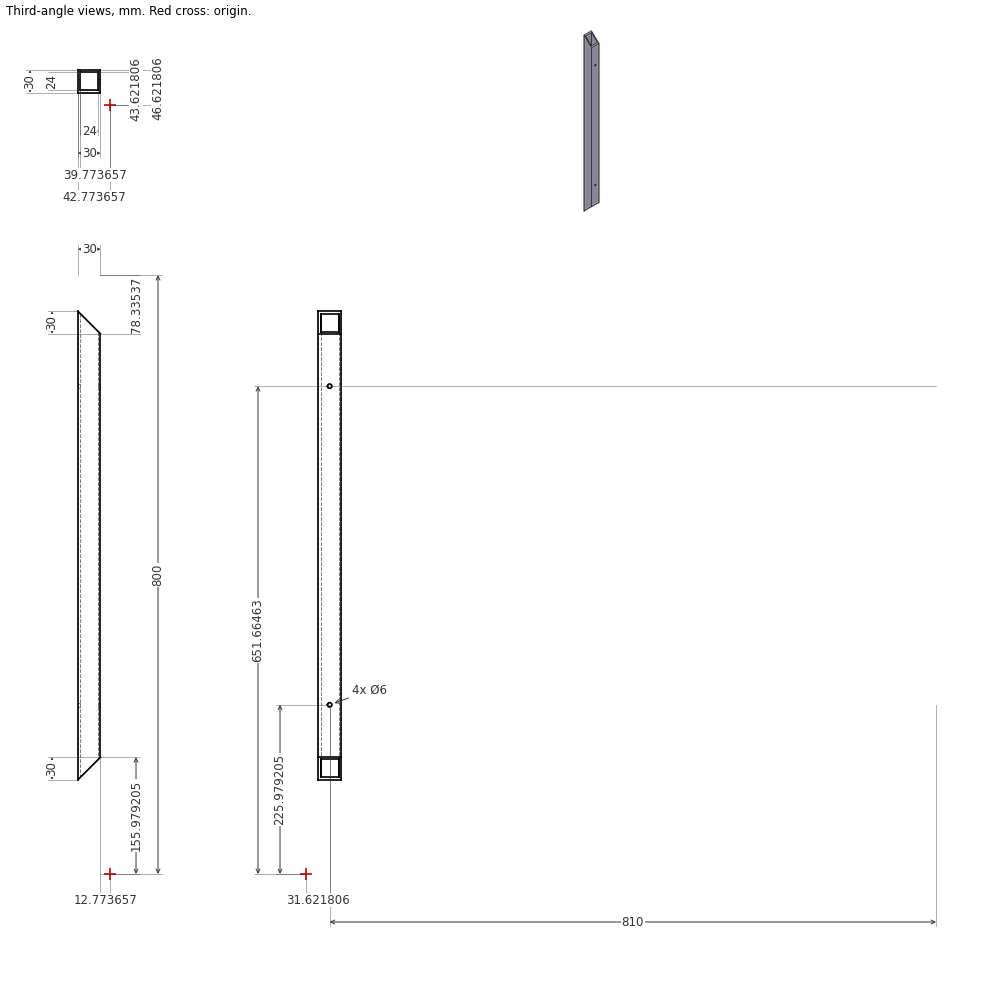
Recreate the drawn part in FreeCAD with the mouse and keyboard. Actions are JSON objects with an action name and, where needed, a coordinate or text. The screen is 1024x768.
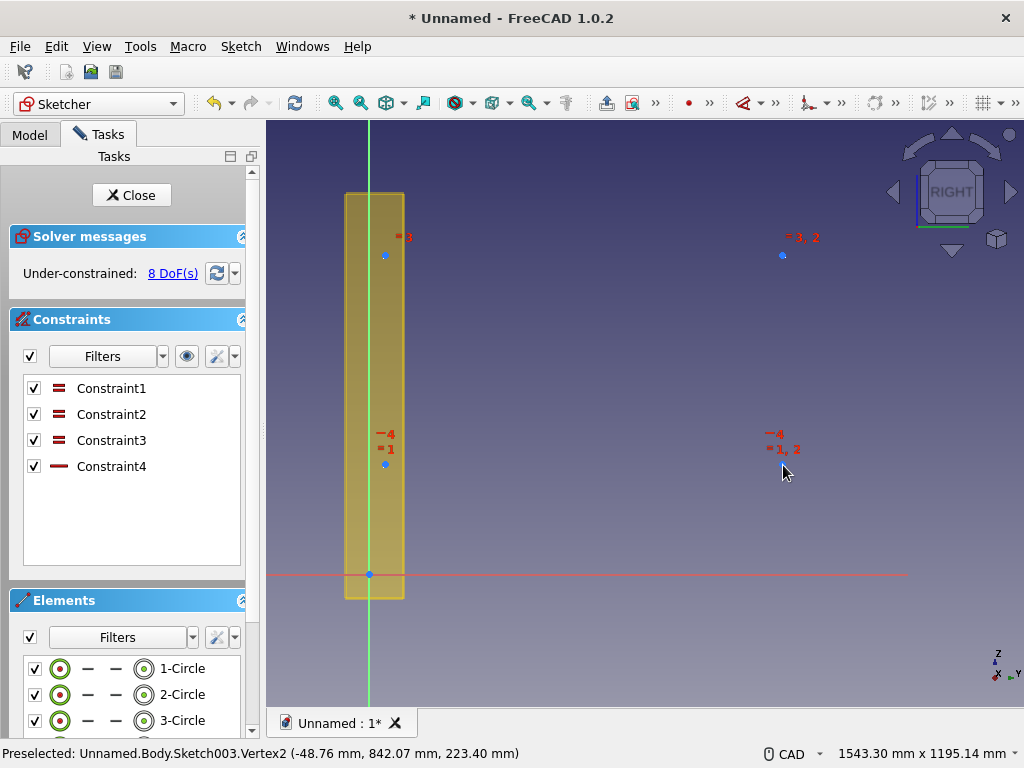
{"action": "left_click", "coordinate": [783, 465]}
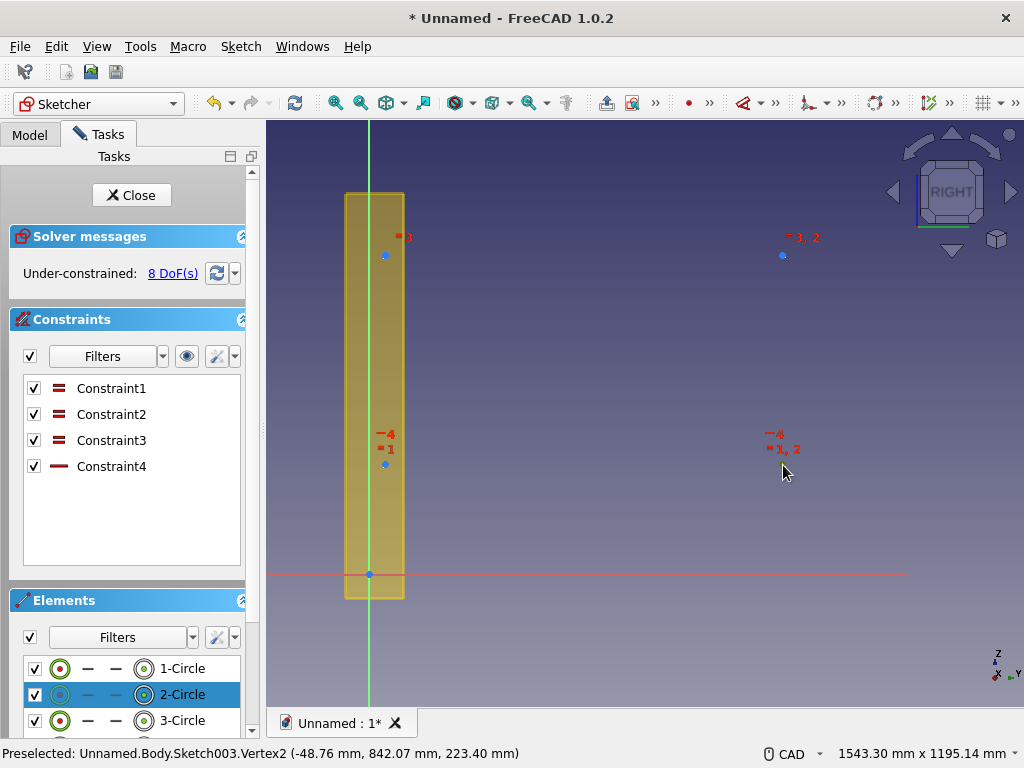
{"action": "left_click", "coordinate": [783, 256]}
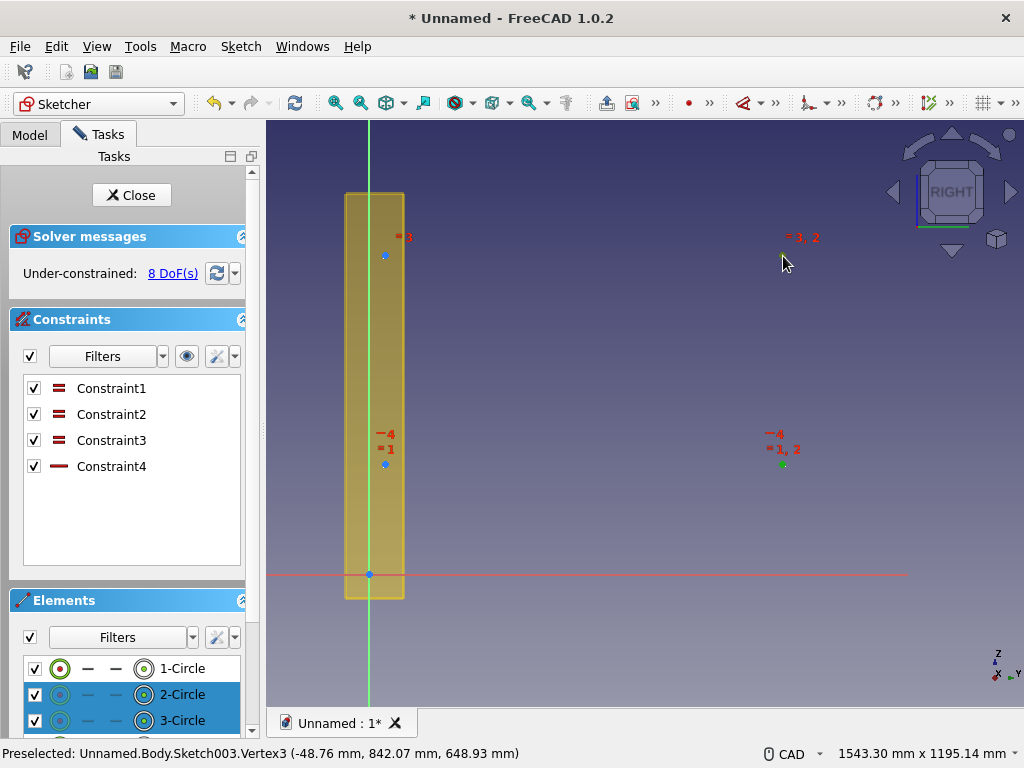
{"action": "key", "text": "v"}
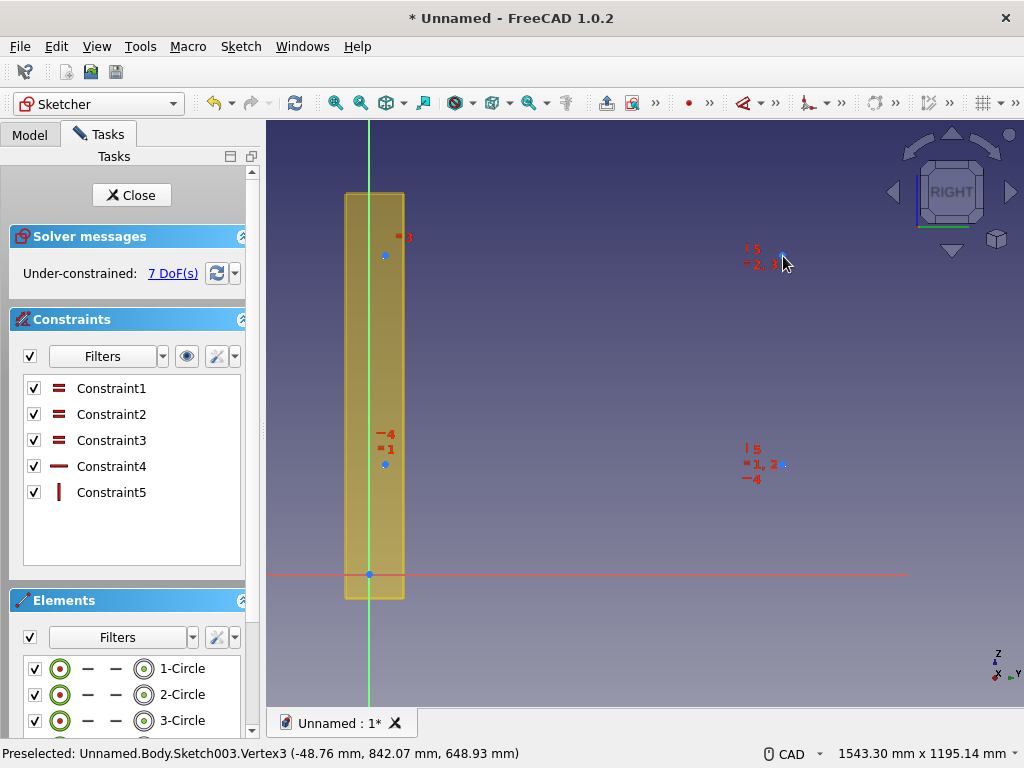
{"action": "left_click", "coordinate": [385, 465]}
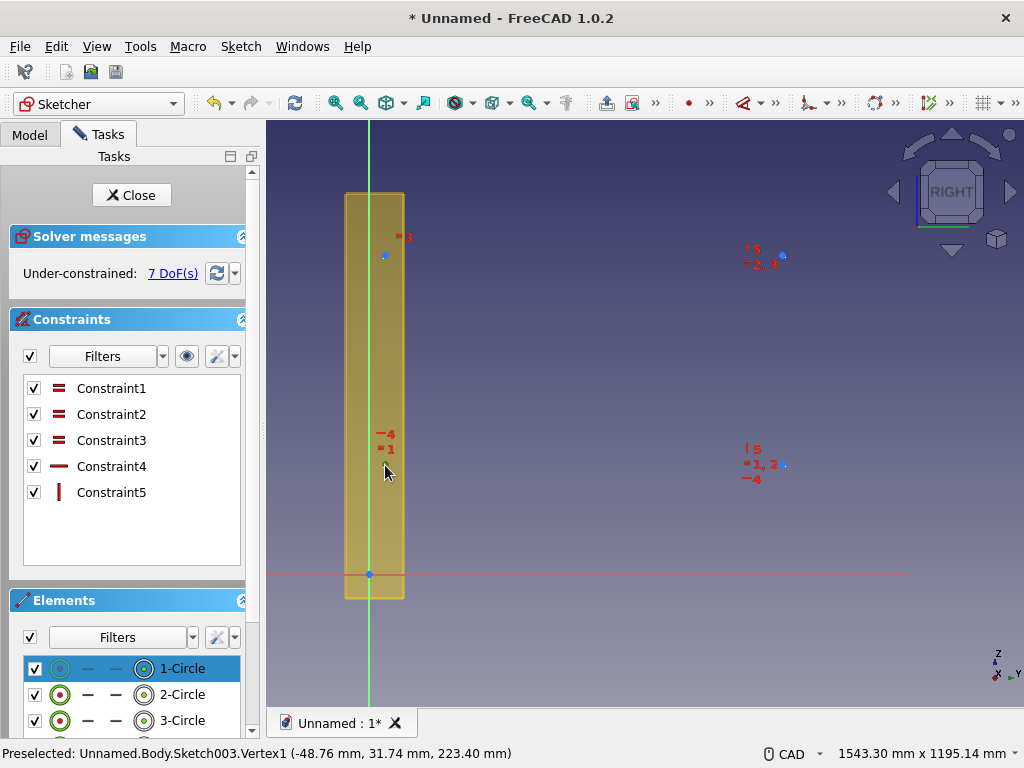
{"action": "left_click", "coordinate": [385, 256]}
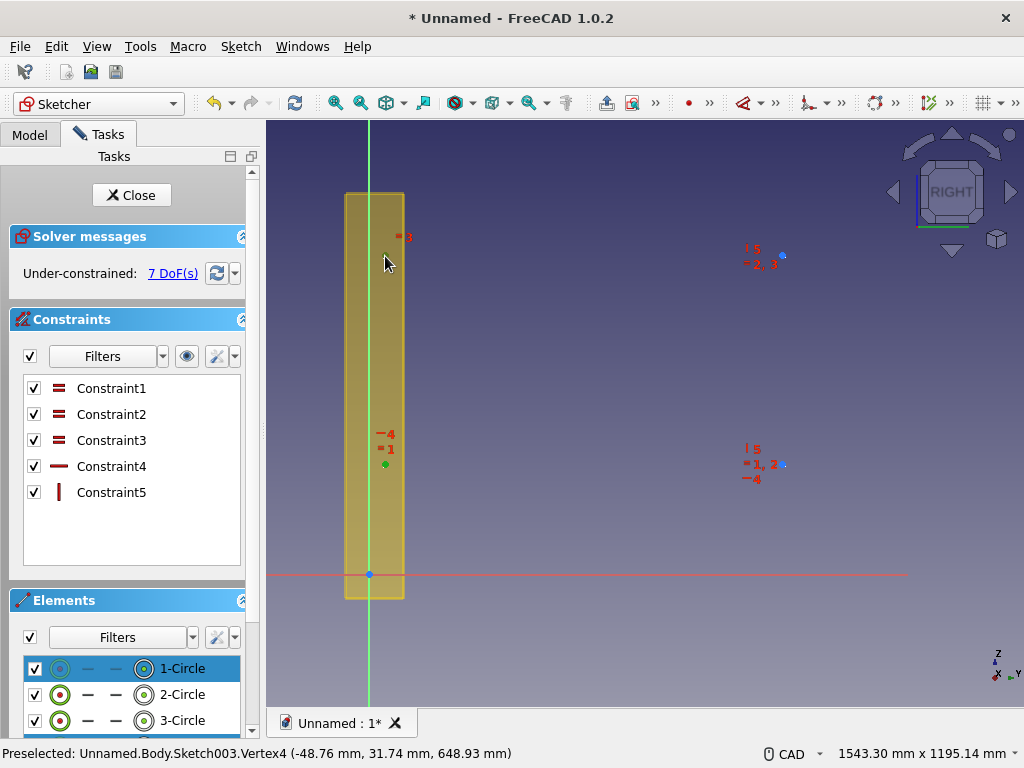
{"action": "key", "text": "v"}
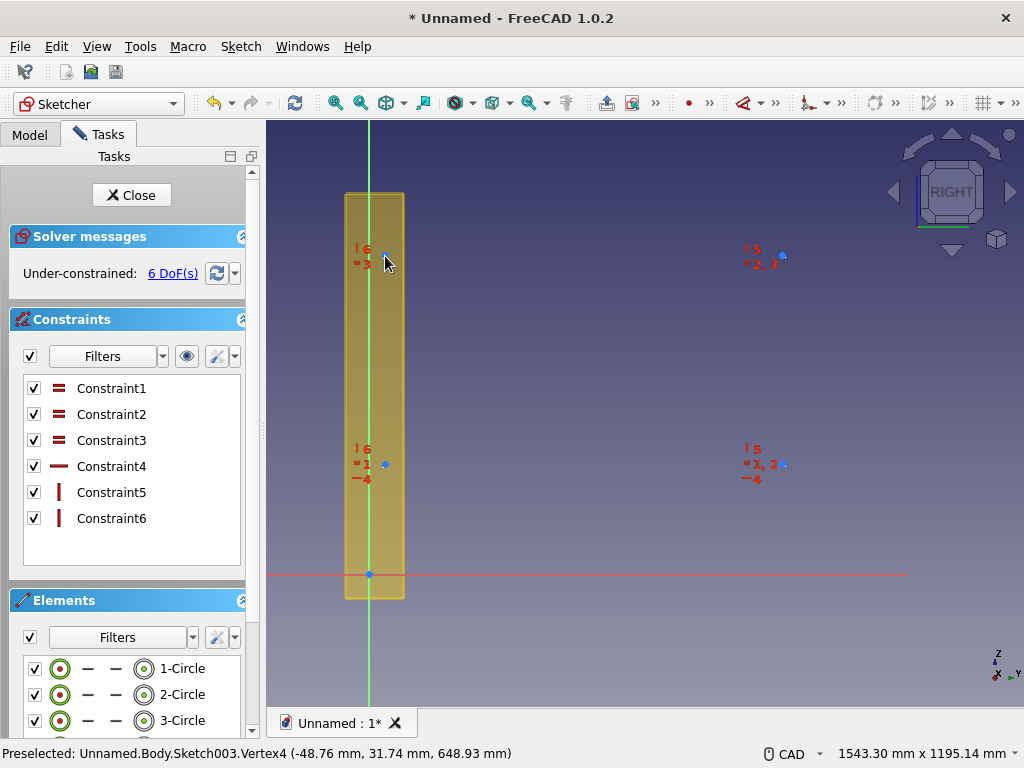
{"action": "left_click", "coordinate": [783, 256]}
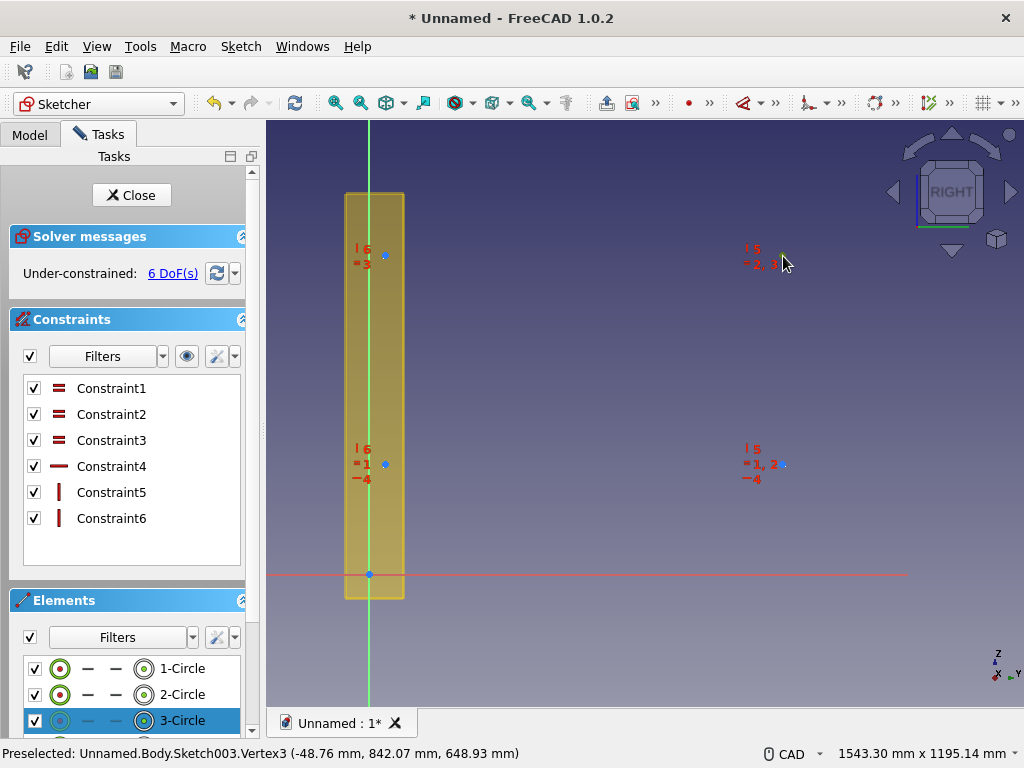
{"action": "left_click", "coordinate": [385, 256]}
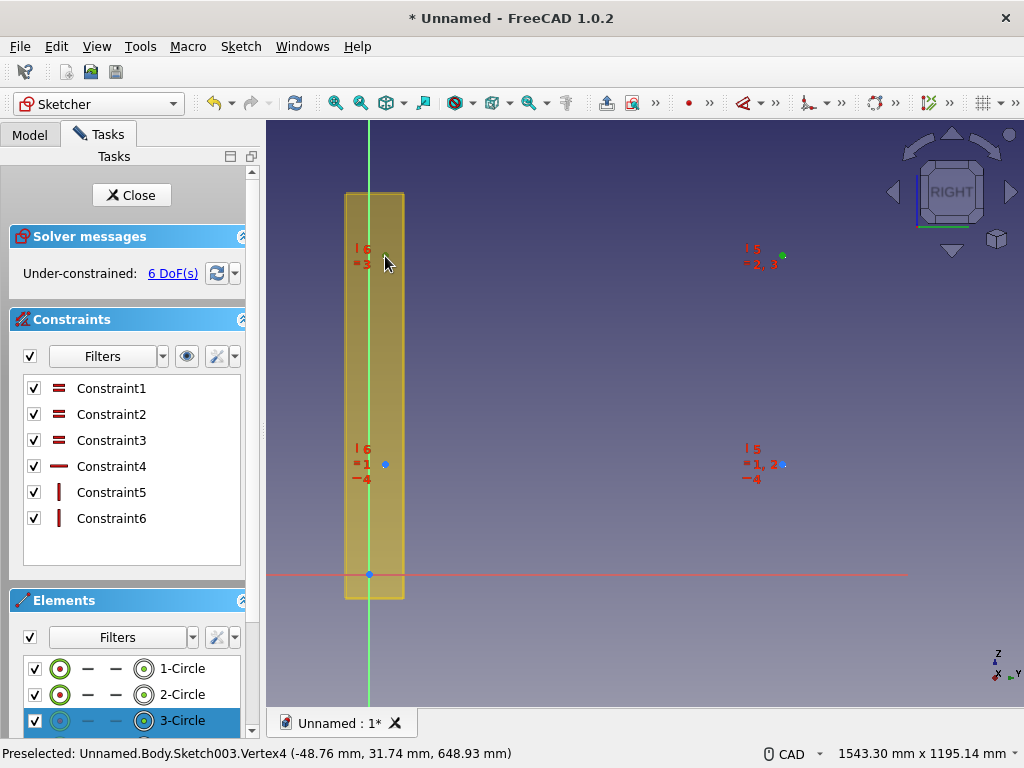
{"action": "key", "text": "h"}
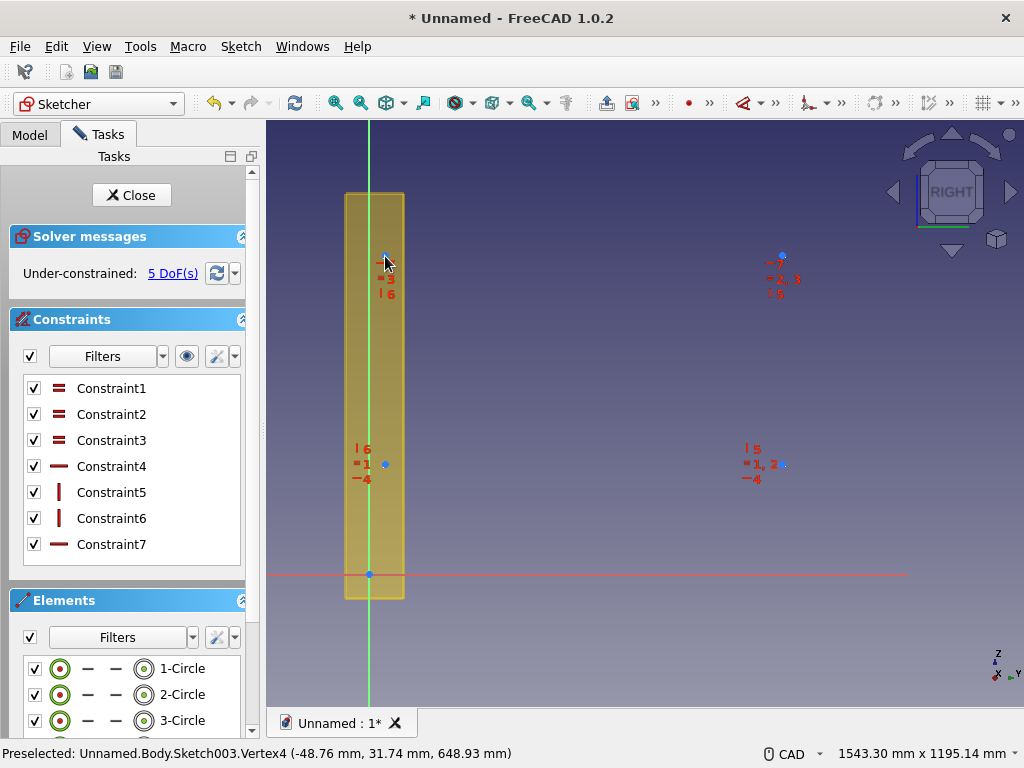
{"action": "left_click", "coordinate": [742, 104]}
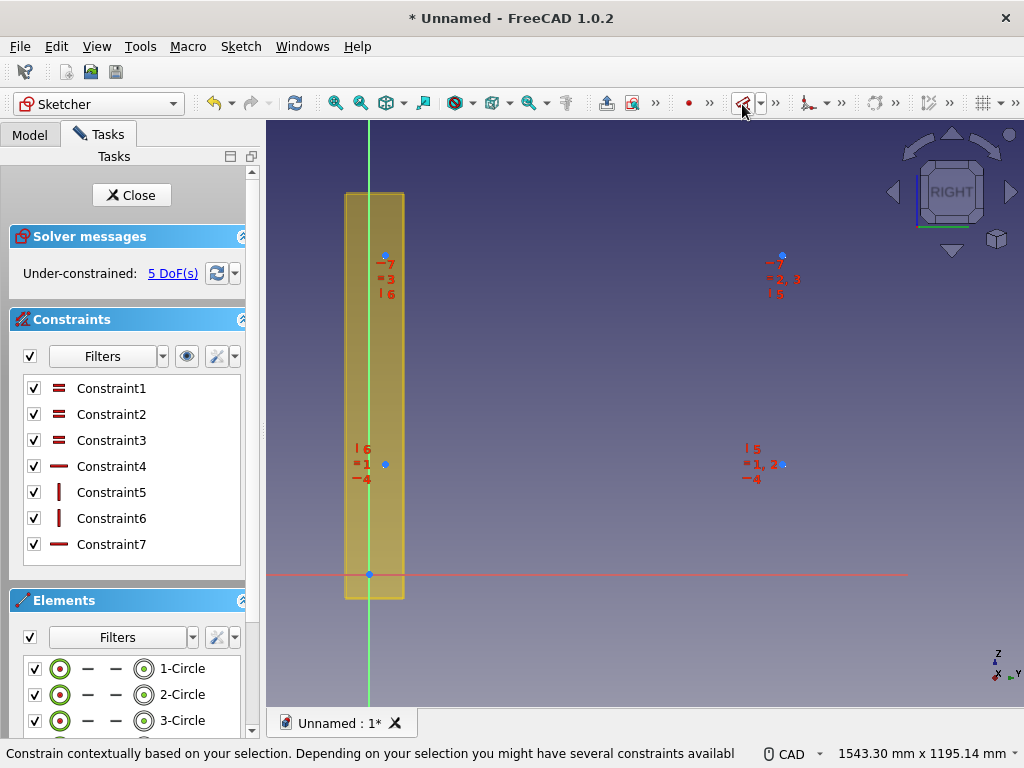
{"action": "scroll", "coordinate": [383, 465], "scroll_direction": "up", "scroll_amount": 14}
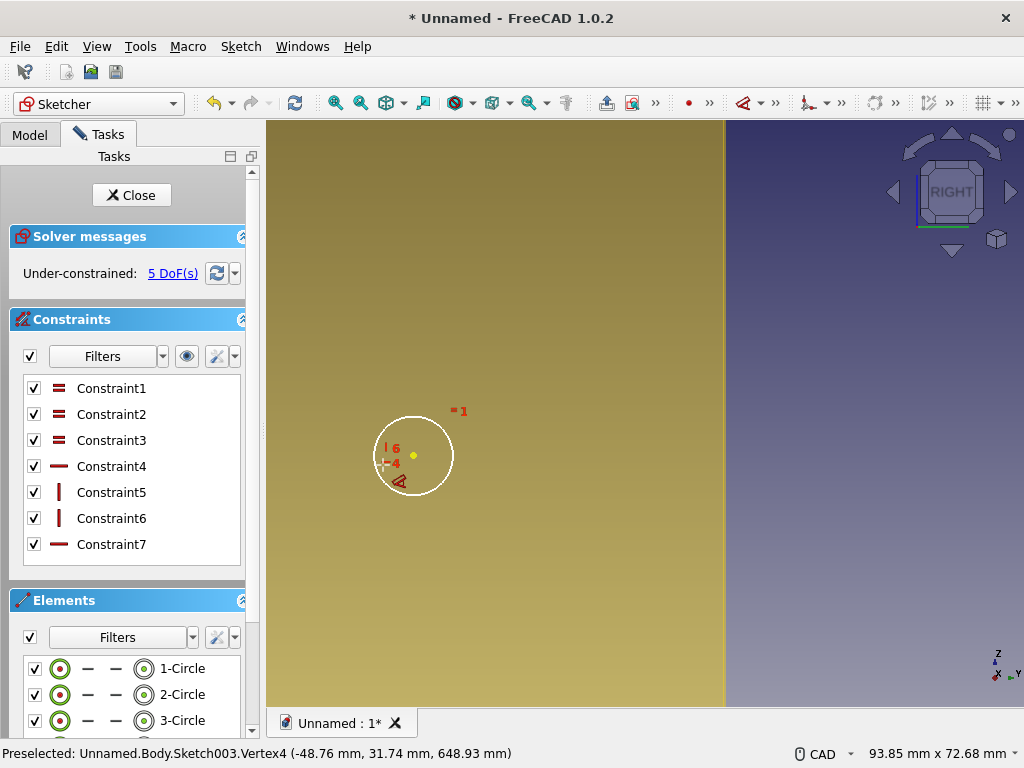
{"action": "left_click", "coordinate": [374, 455]}
{"action": "left_click", "coordinate": [342, 454]}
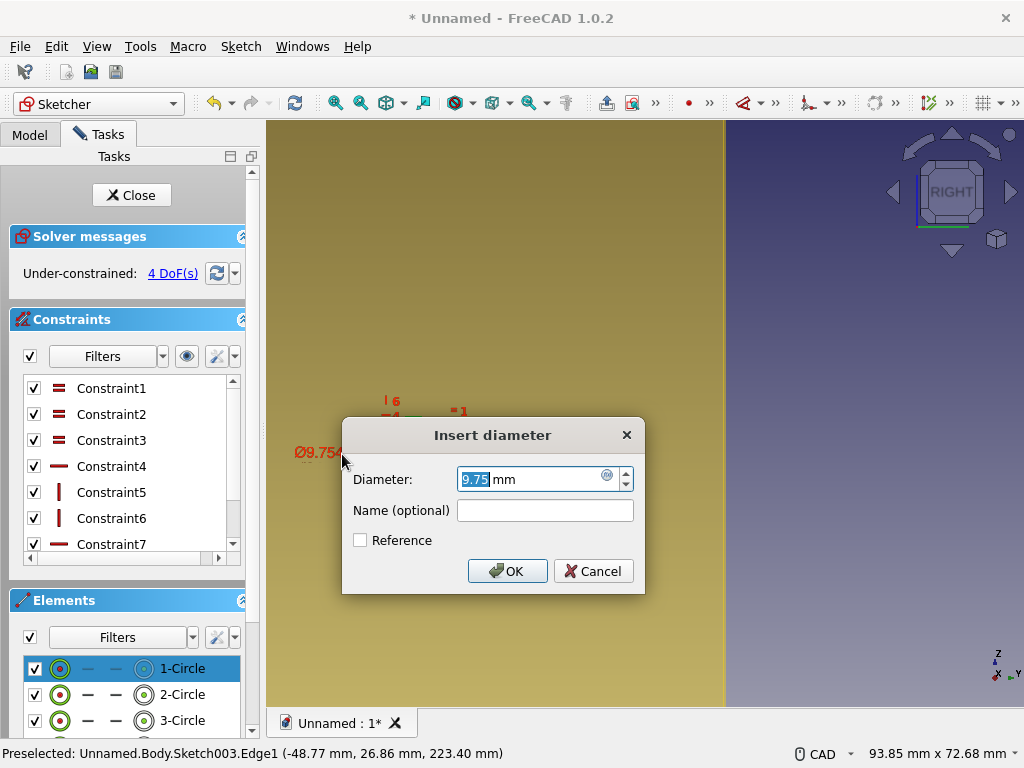
{"action": "type", "text": "6"}
{"action": "key", "text": "Return"}